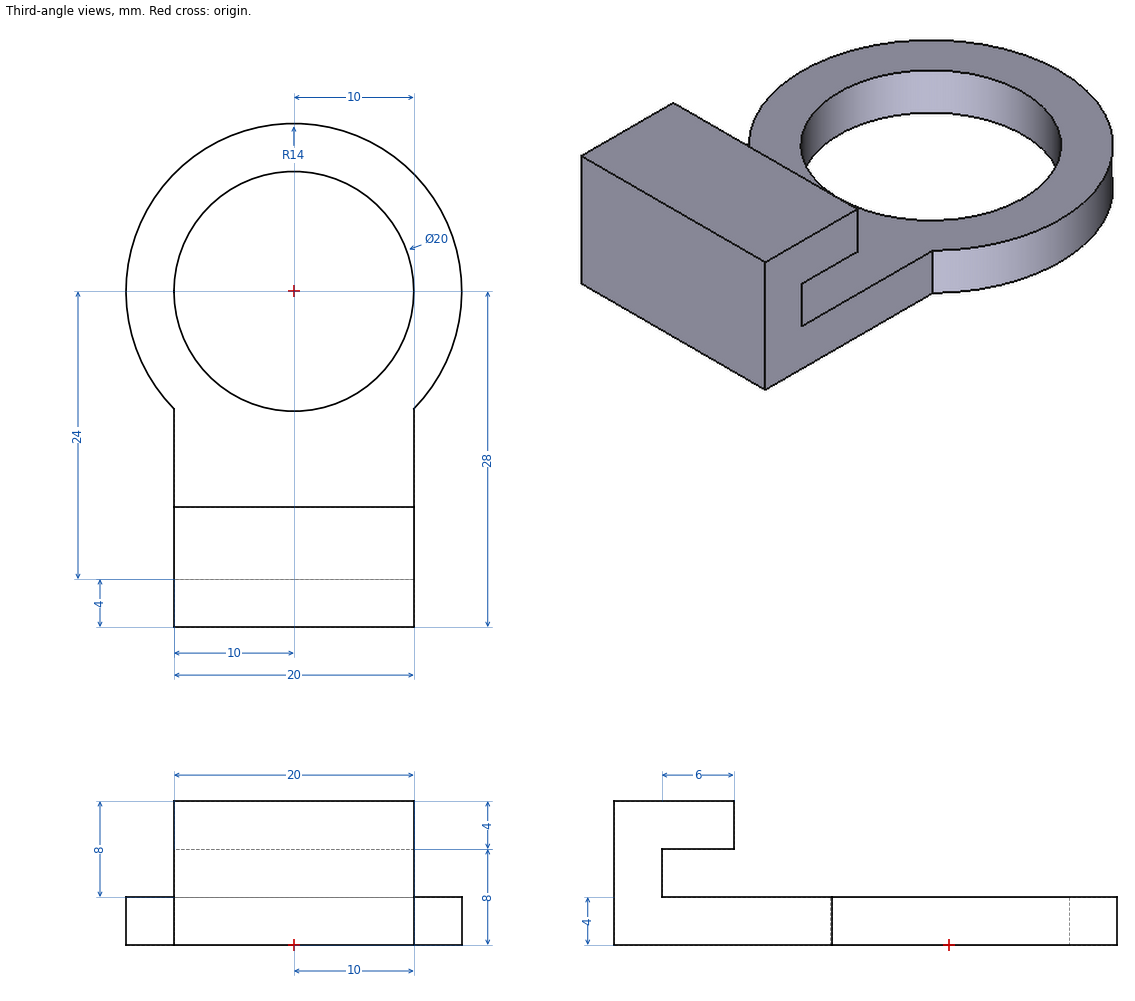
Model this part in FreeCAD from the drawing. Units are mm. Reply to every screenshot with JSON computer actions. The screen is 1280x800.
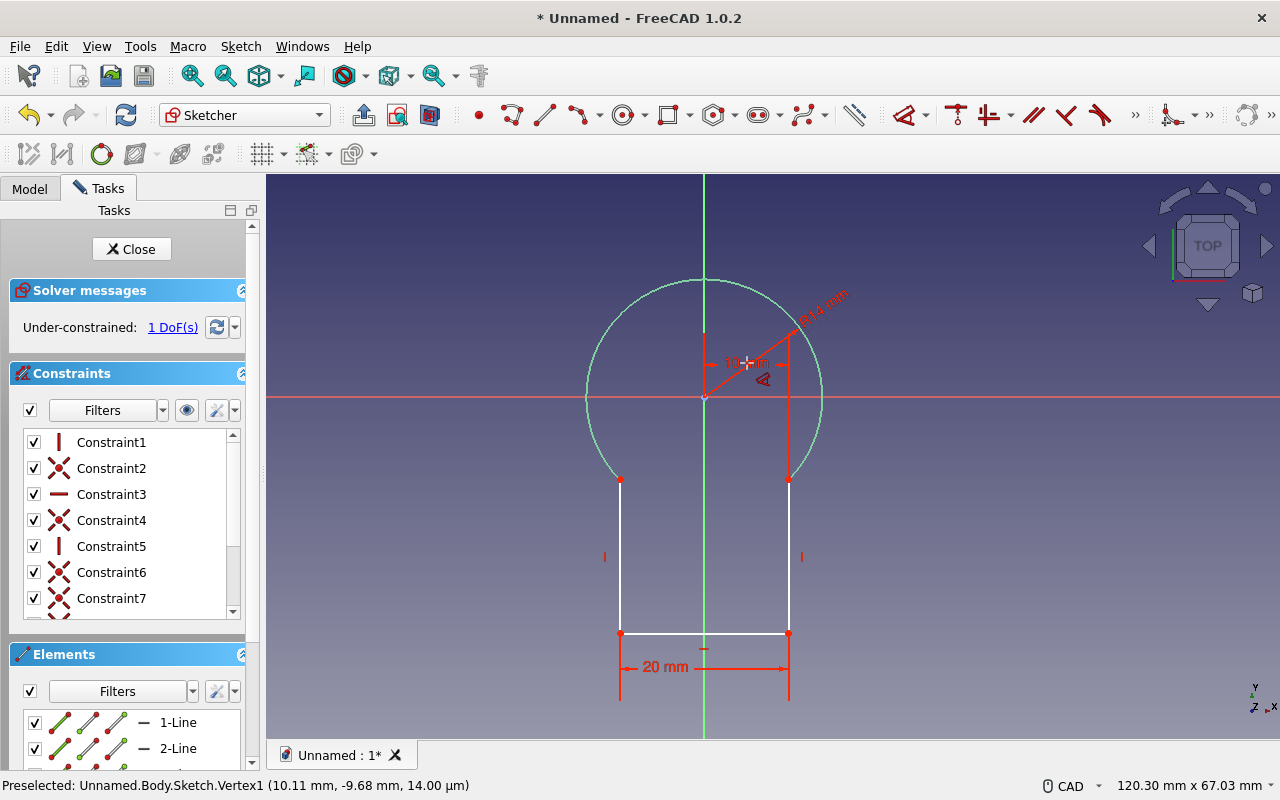
{"action": "left_click", "coordinate": [789, 634]}
{"action": "left_click", "coordinate": [823, 516]}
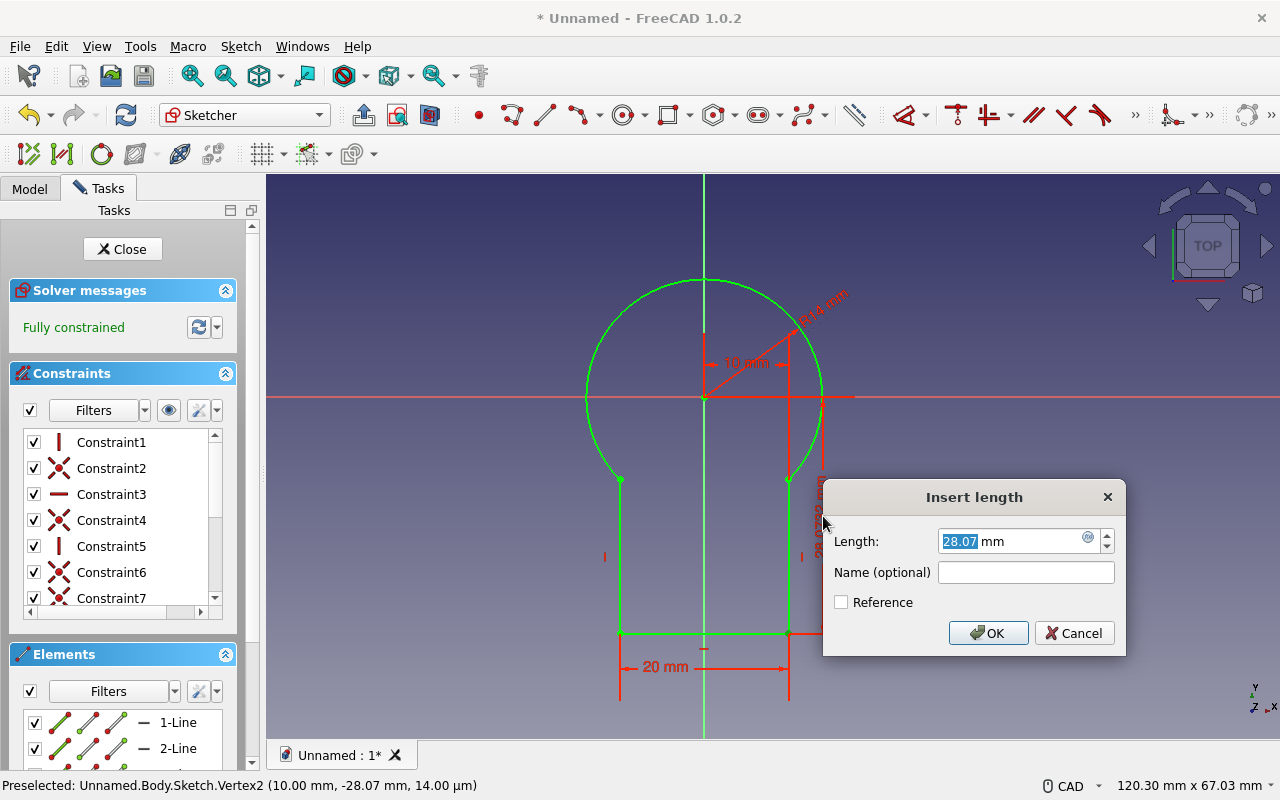
{"action": "type", "text": "28"}
{"action": "key", "text": "Return"}
{"action": "key", "text": "Escape"}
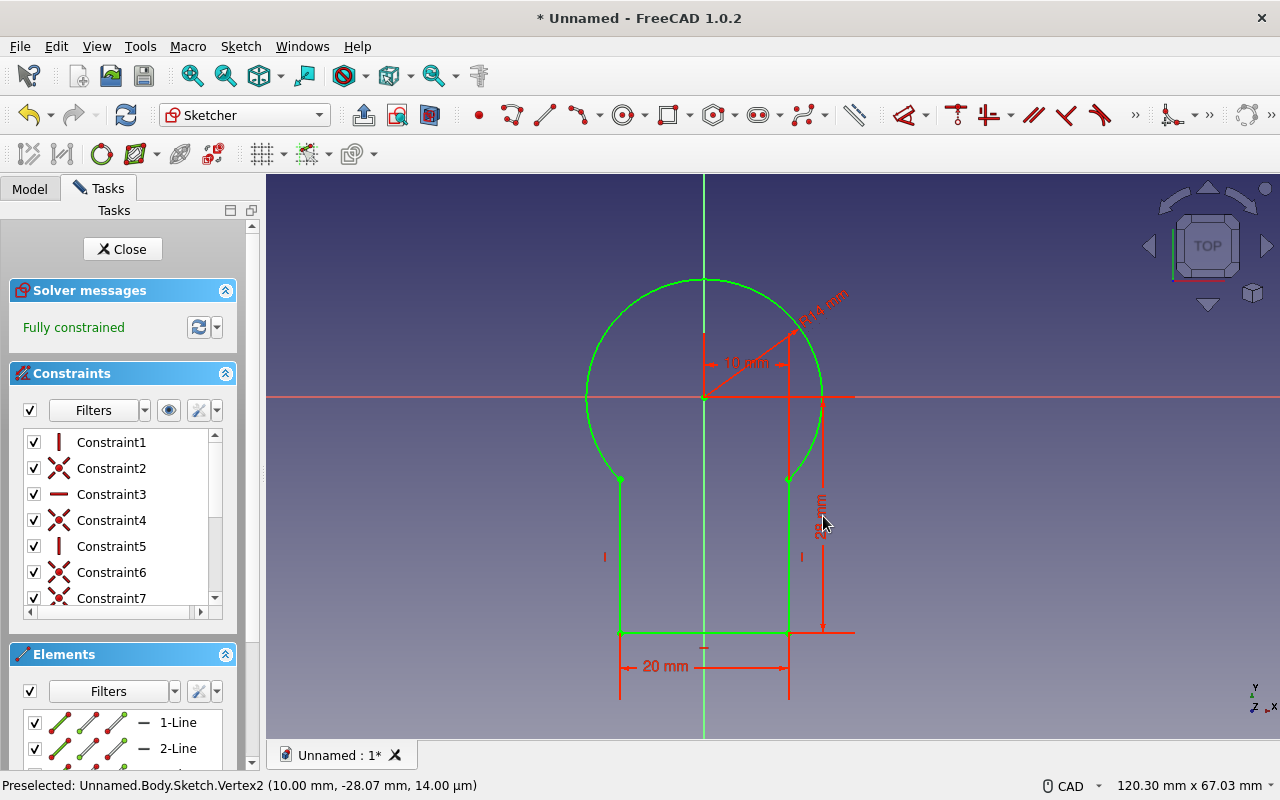
{"action": "left_click", "coordinate": [123, 249]}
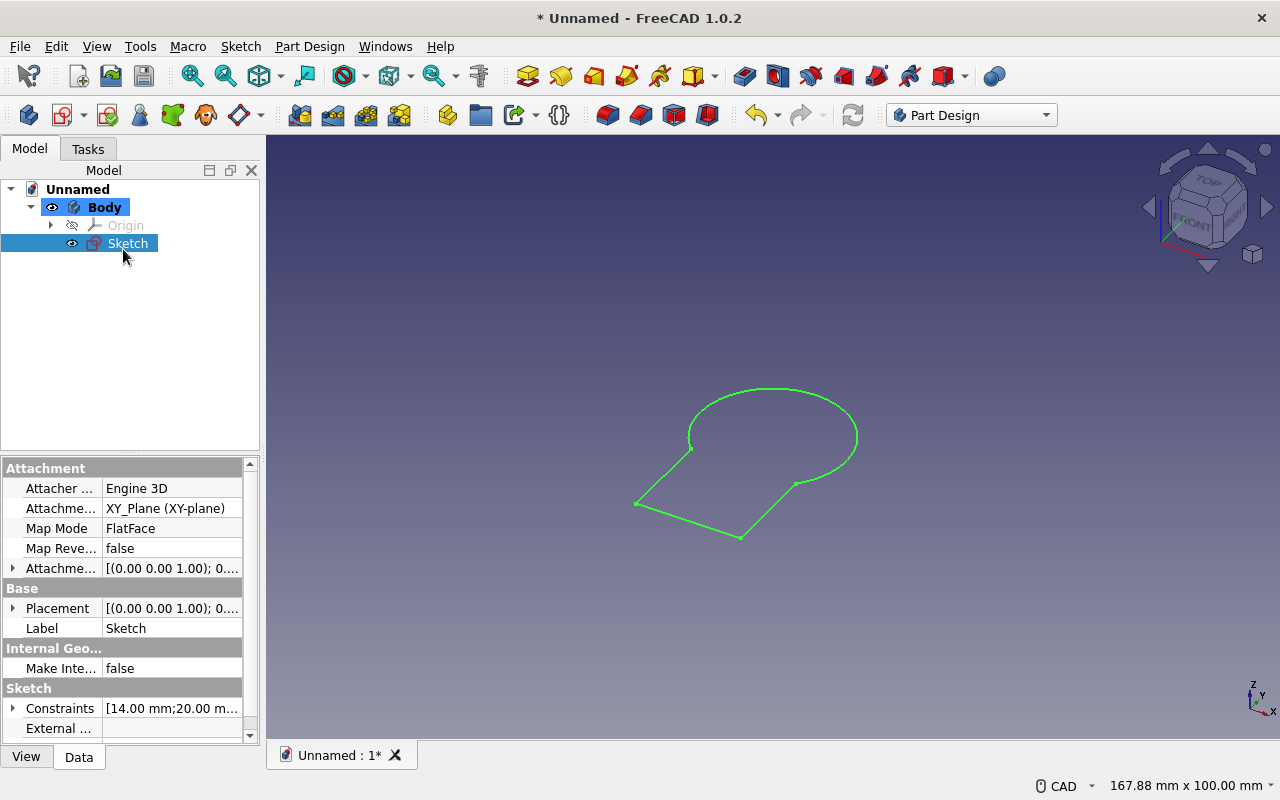
{"action": "left_click", "coordinate": [528, 76]}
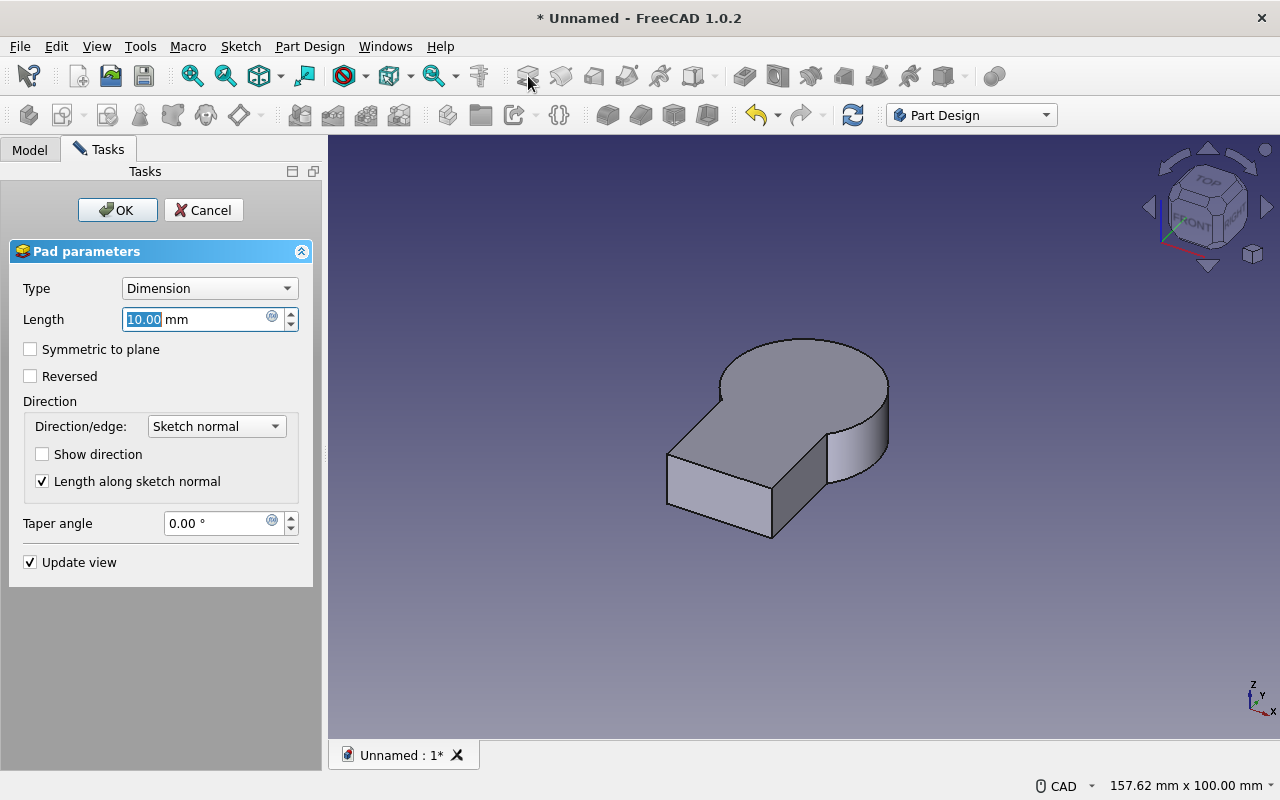
{"action": "type", "text": "4"}
{"action": "key", "text": "Tab"}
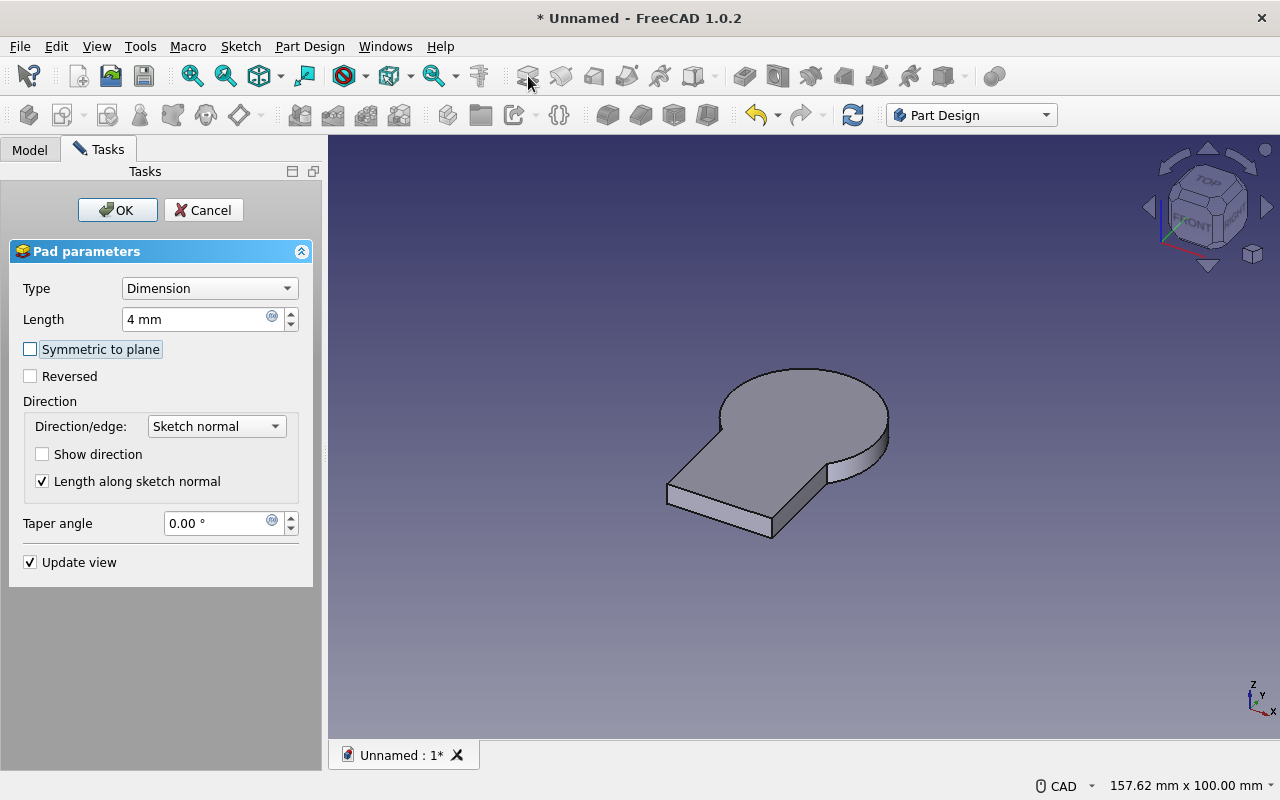
{"action": "left_click", "coordinate": [118, 210]}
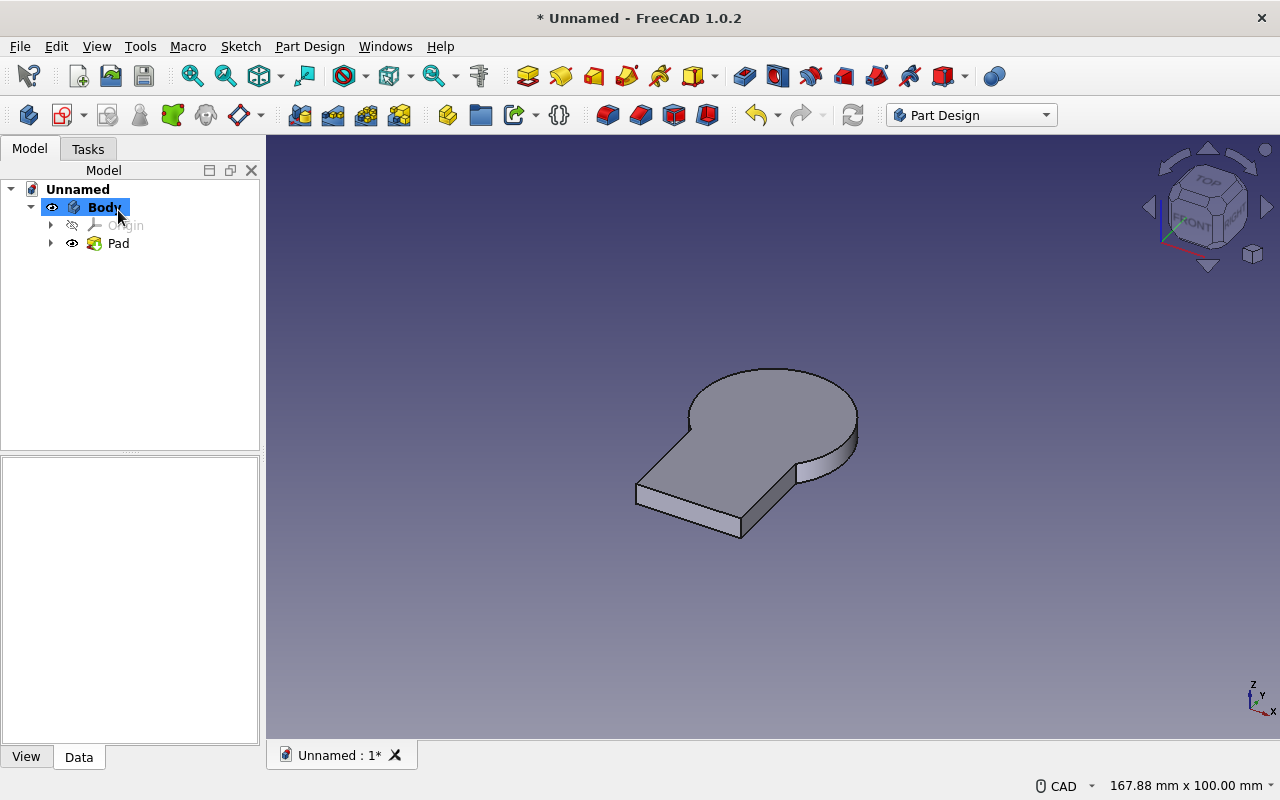
{"action": "left_click", "coordinate": [193, 76]}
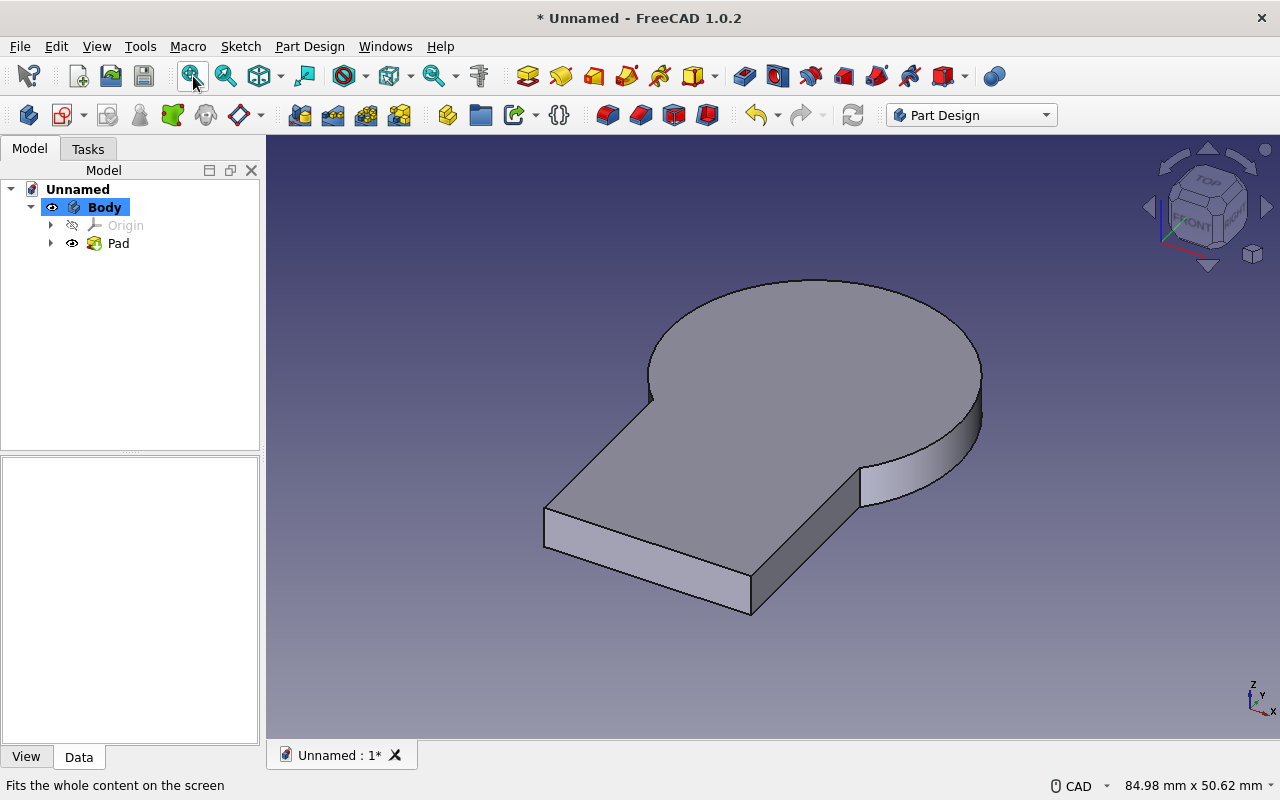
{"action": "left_click", "coordinate": [809, 381]}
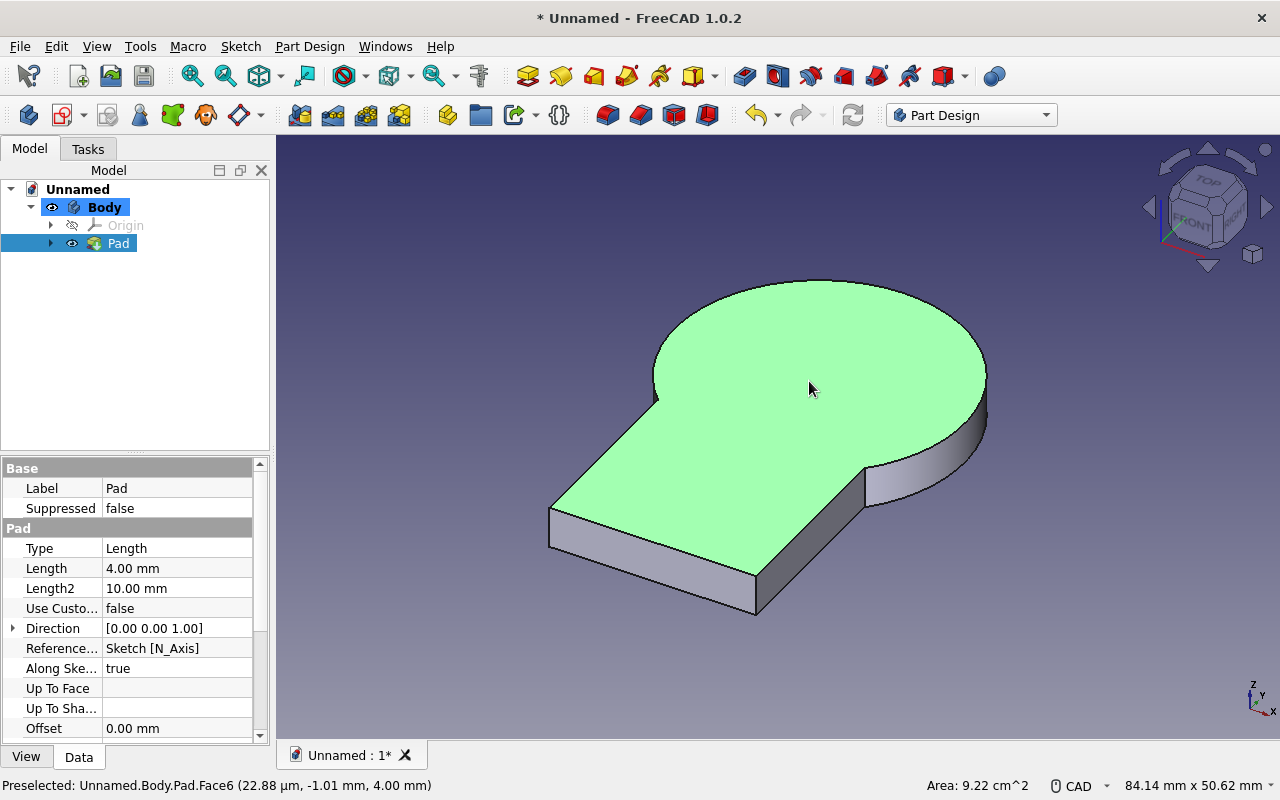
{"action": "left_click", "coordinate": [62, 116]}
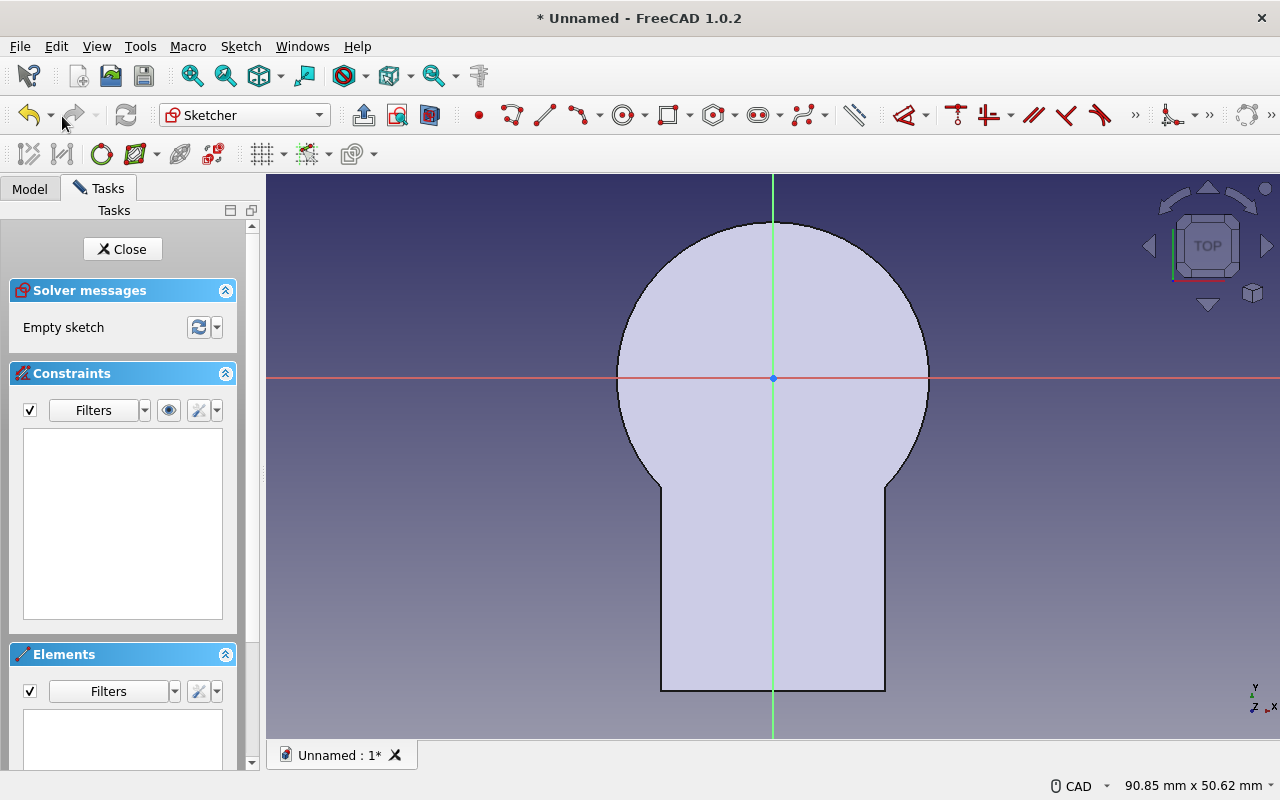
{"action": "scroll", "coordinate": [395, 202], "scroll_direction": "down", "scroll_amount": 1}